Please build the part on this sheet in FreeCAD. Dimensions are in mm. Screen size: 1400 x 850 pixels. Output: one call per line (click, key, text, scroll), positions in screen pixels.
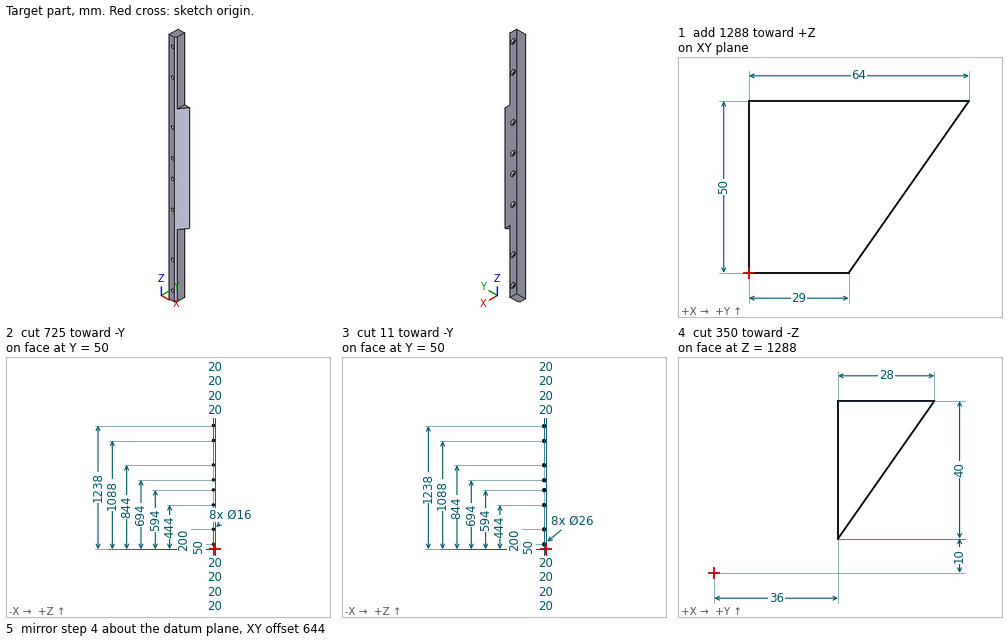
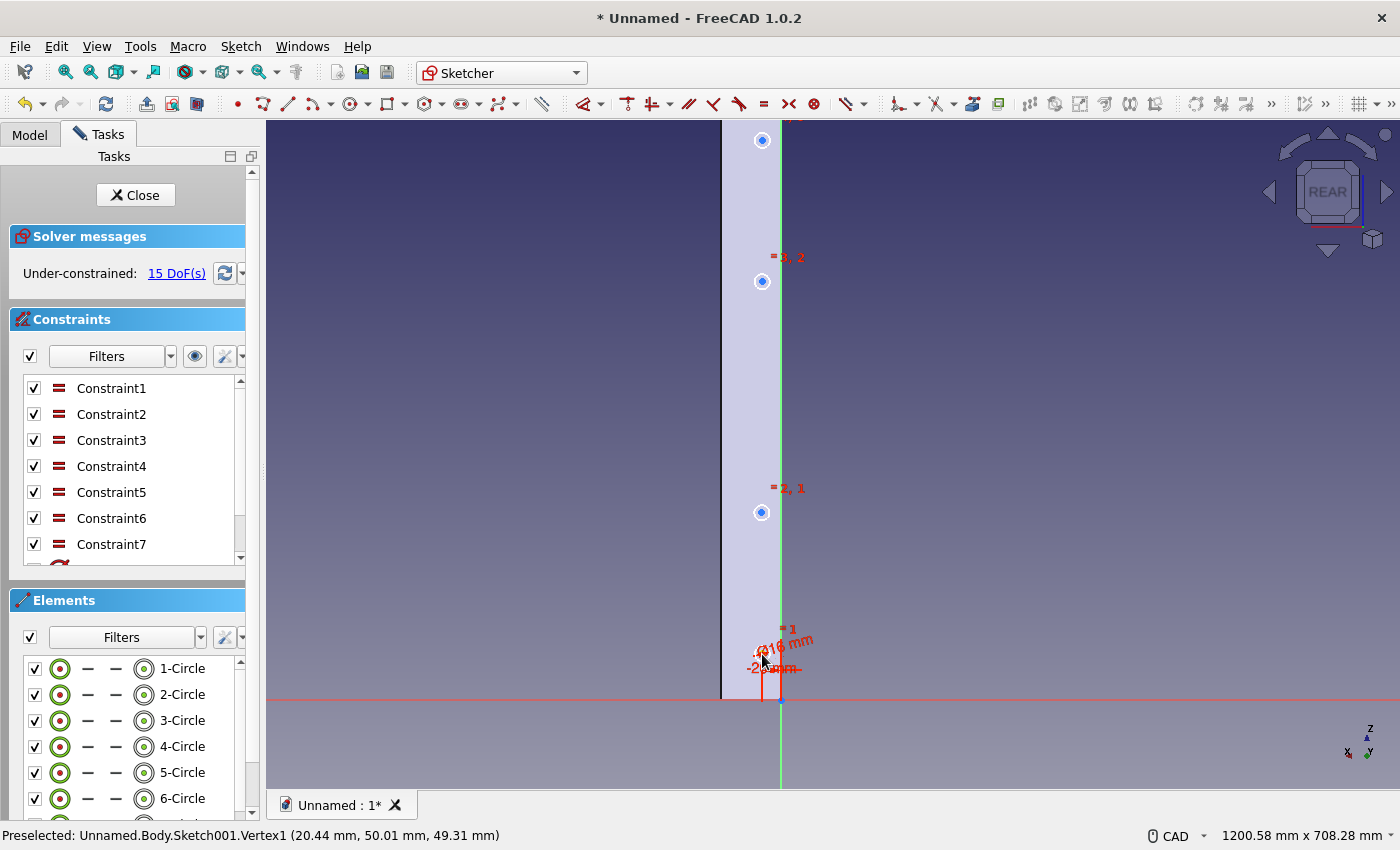
click(762, 654)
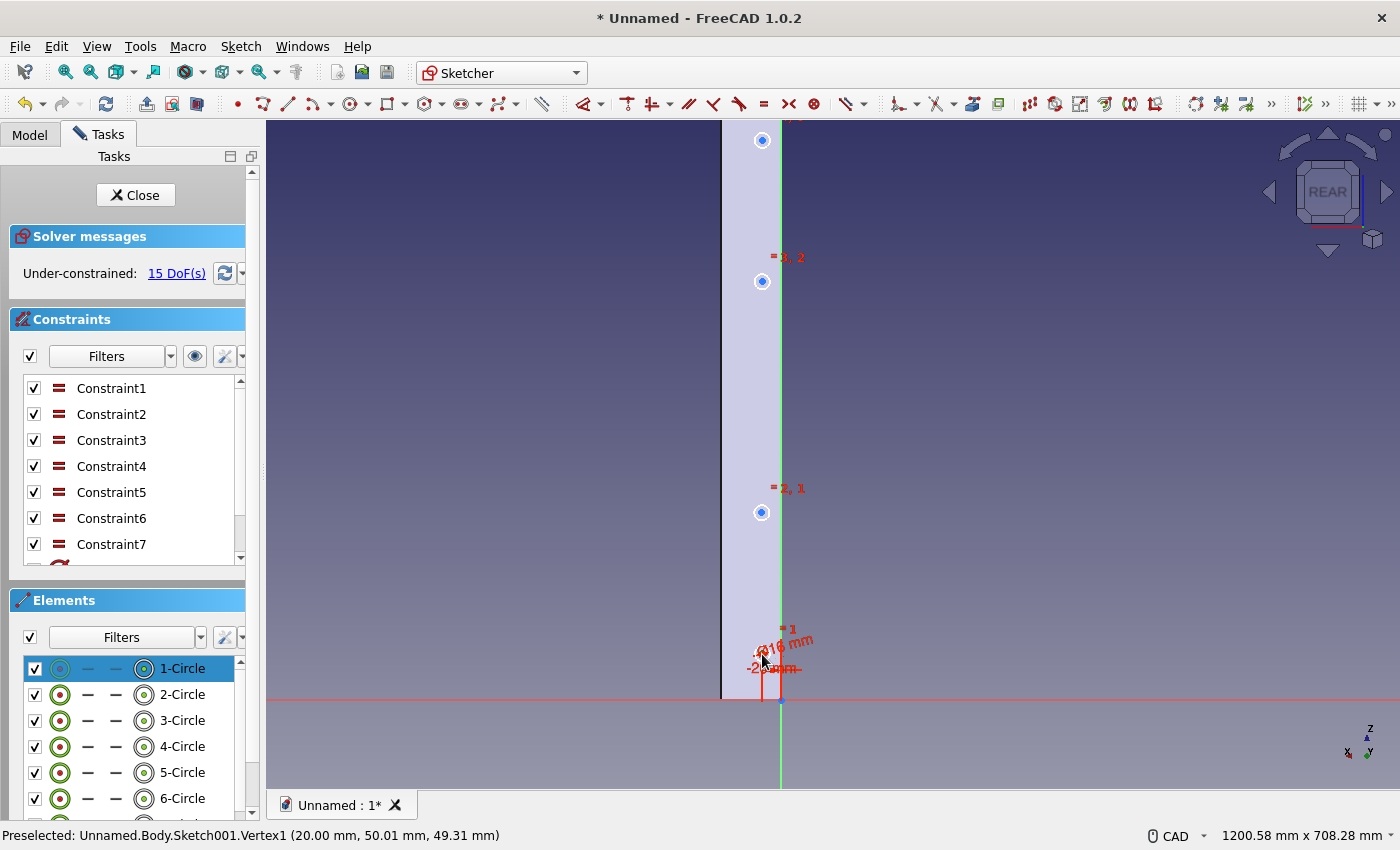
click(600, 104)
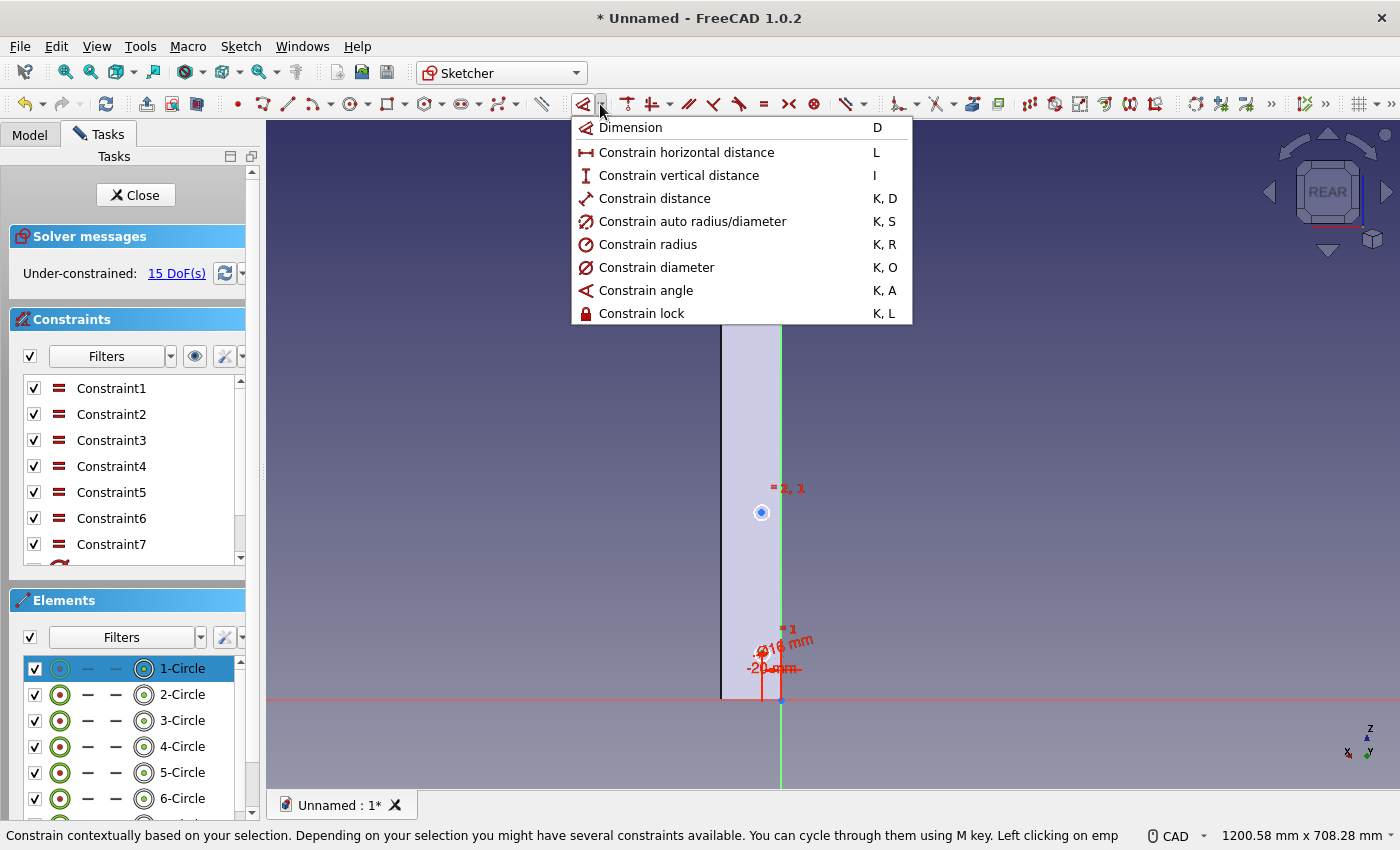
click(742, 176)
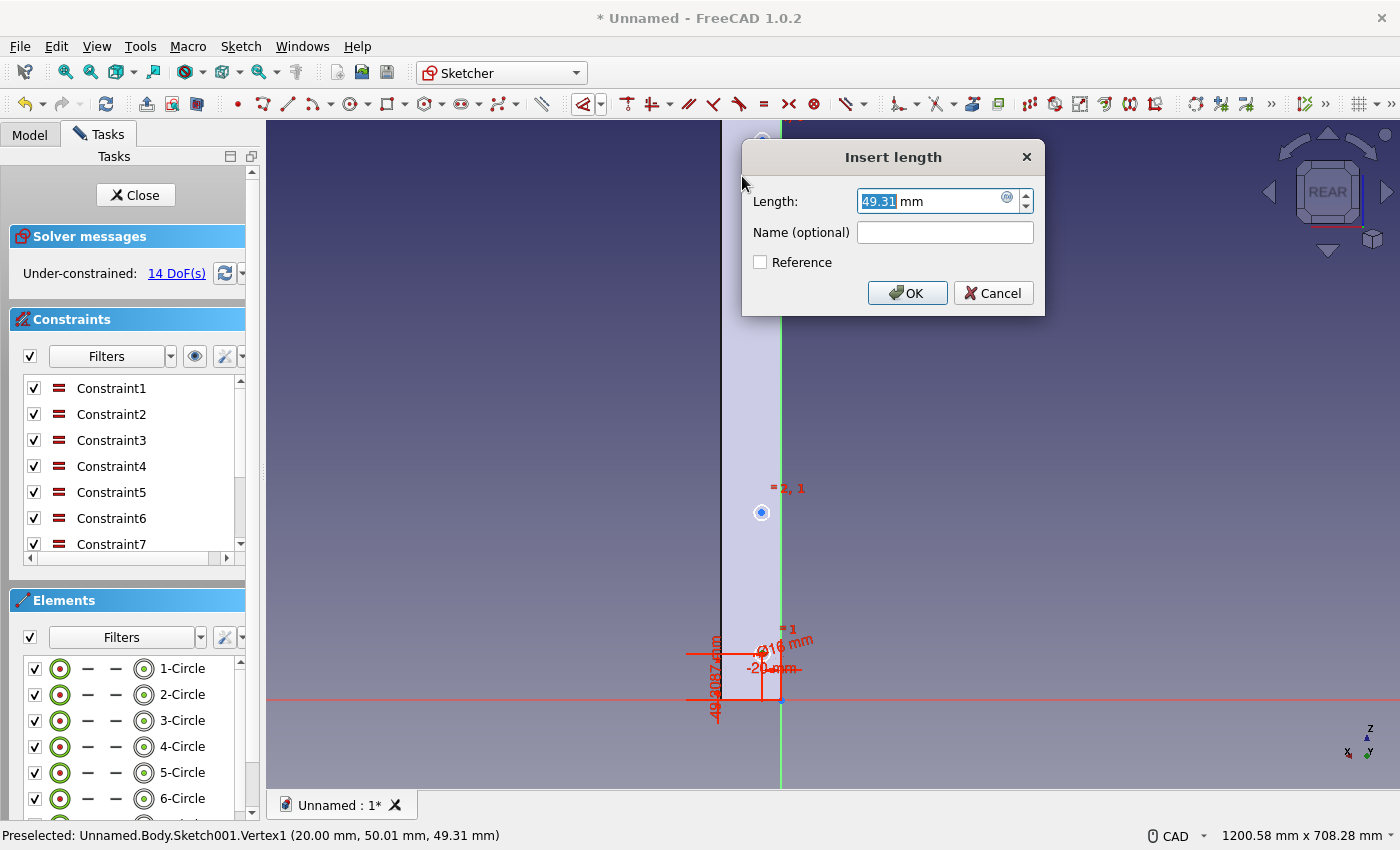
text(50)
key(Return)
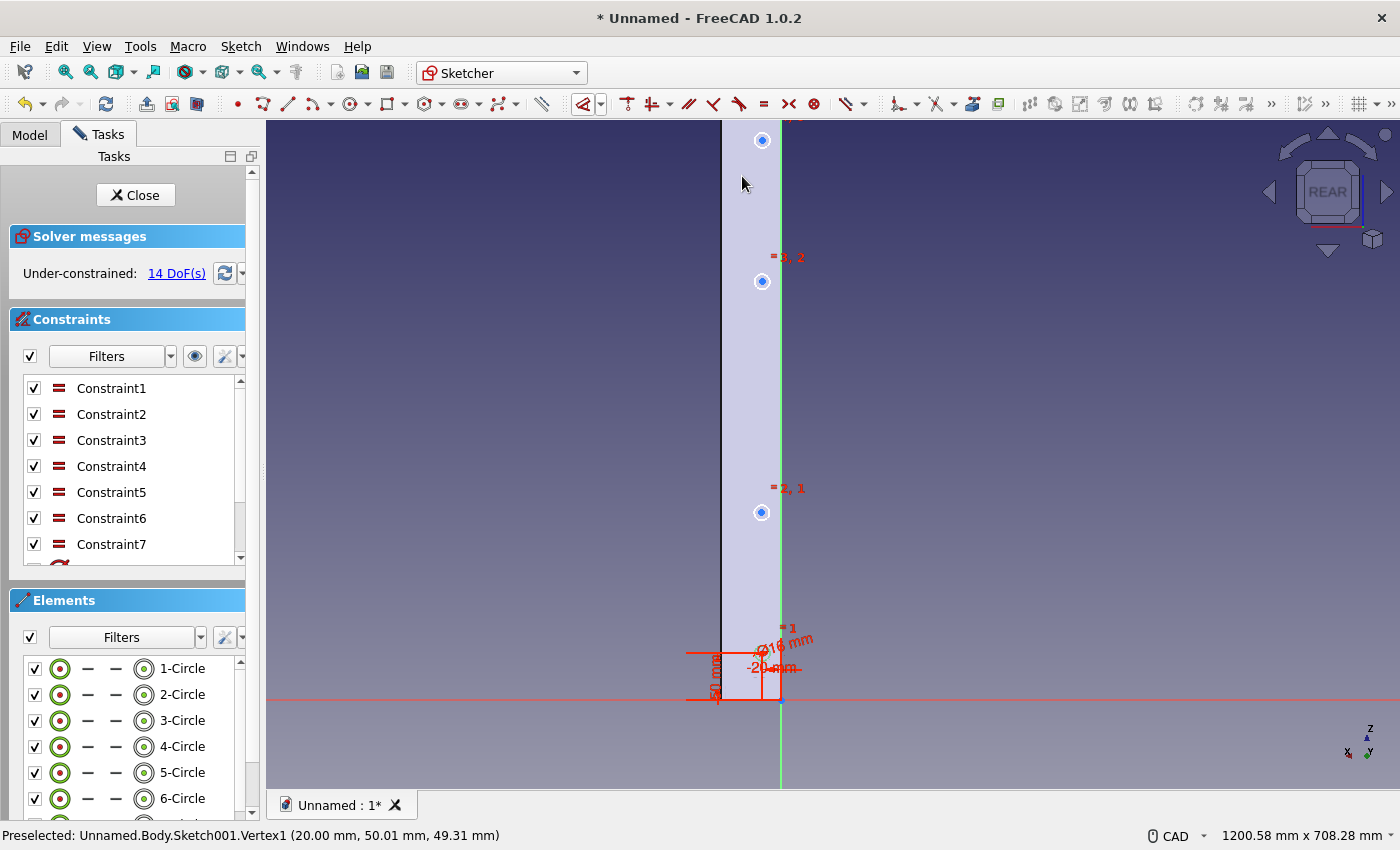
scroll(762, 513, up, 4)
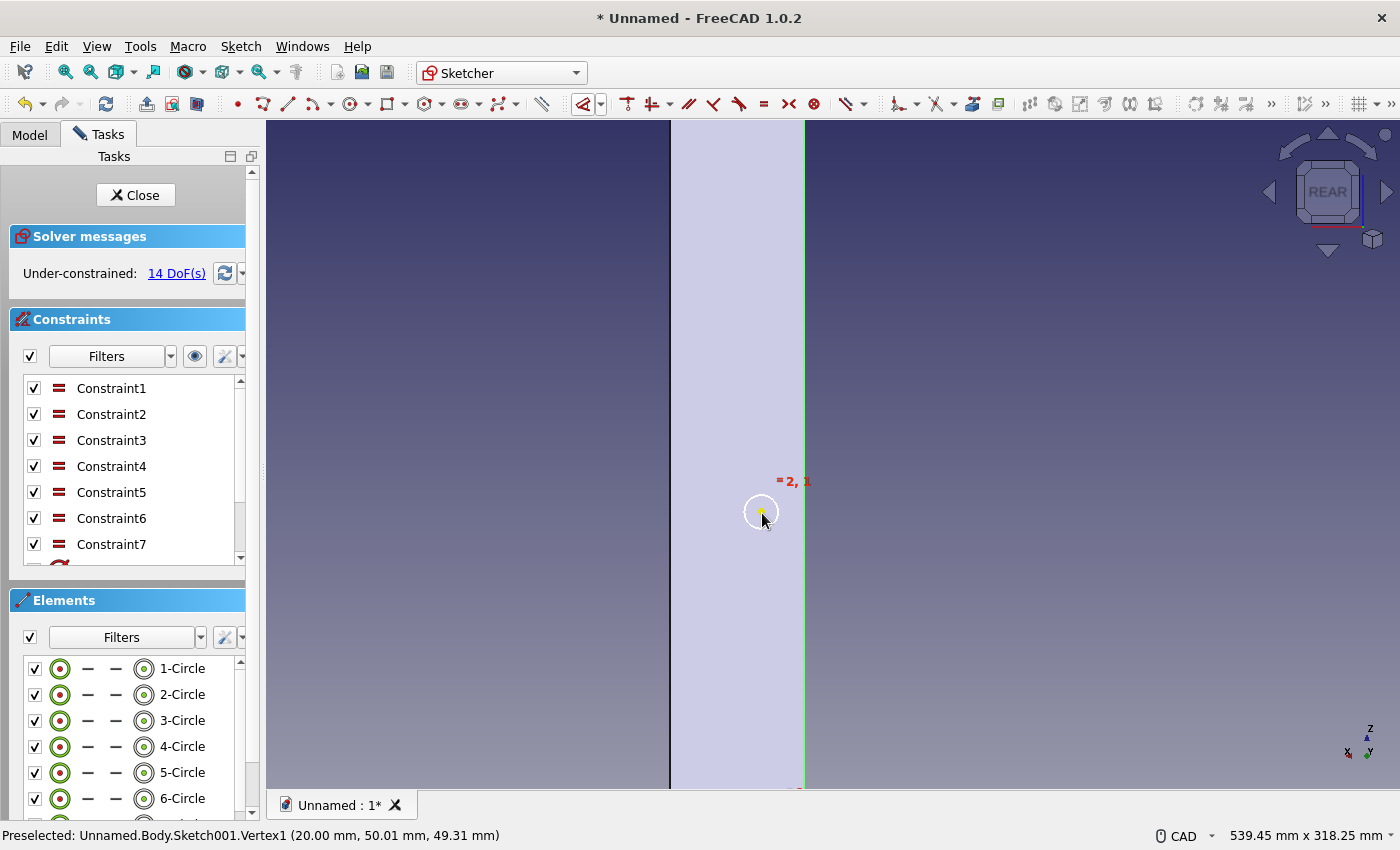
click(761, 512)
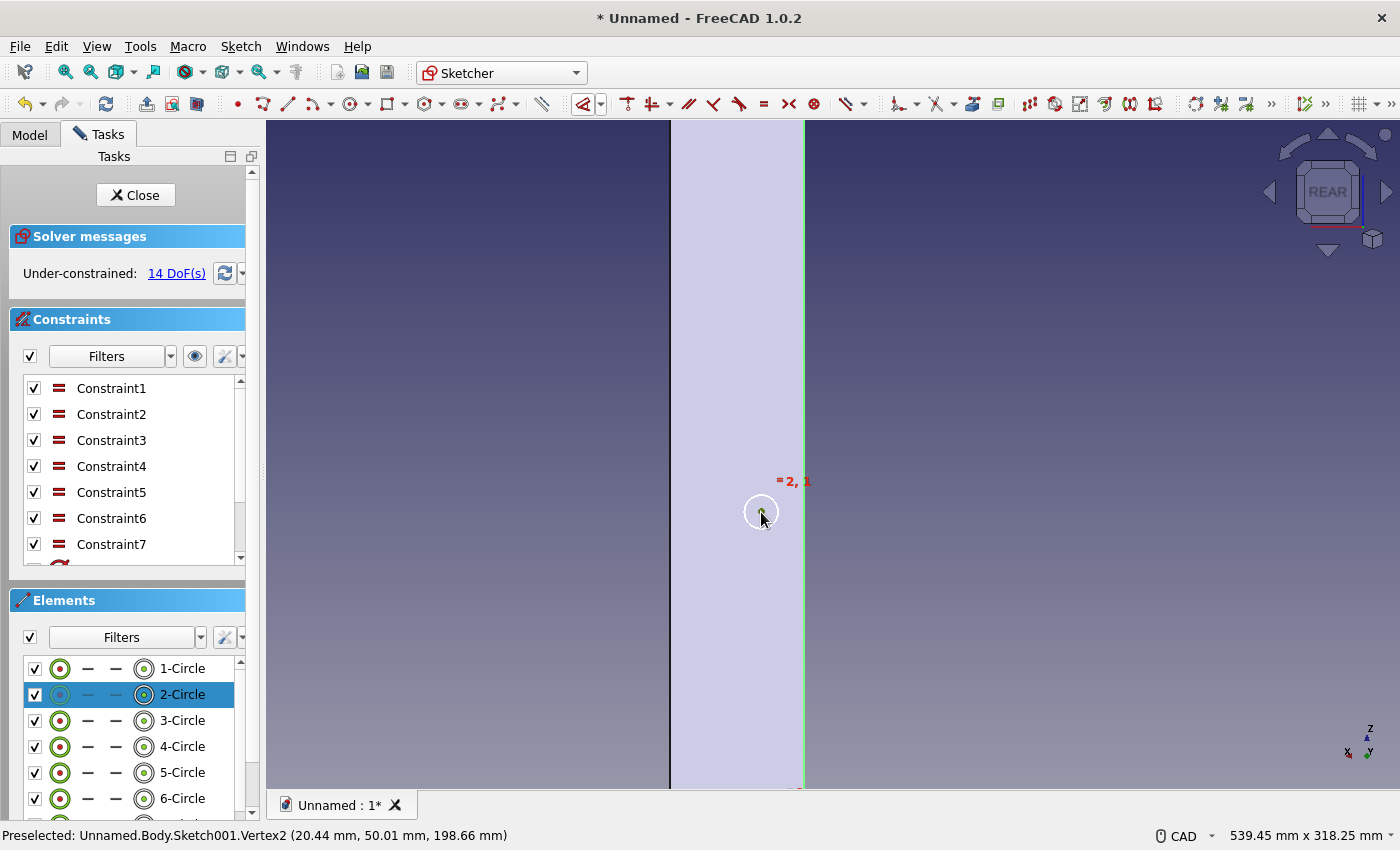
key(l)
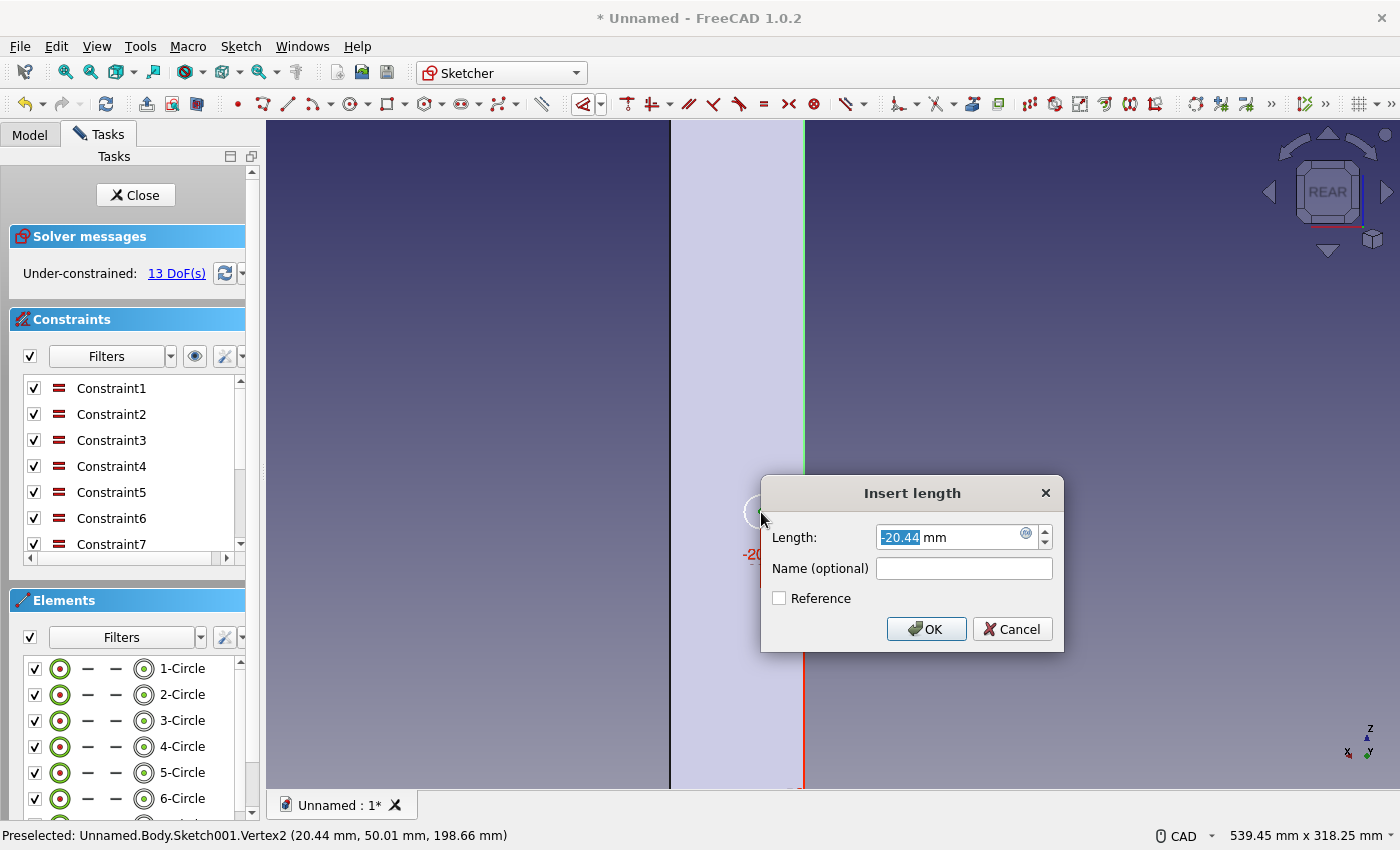
text(-20)
key(Return)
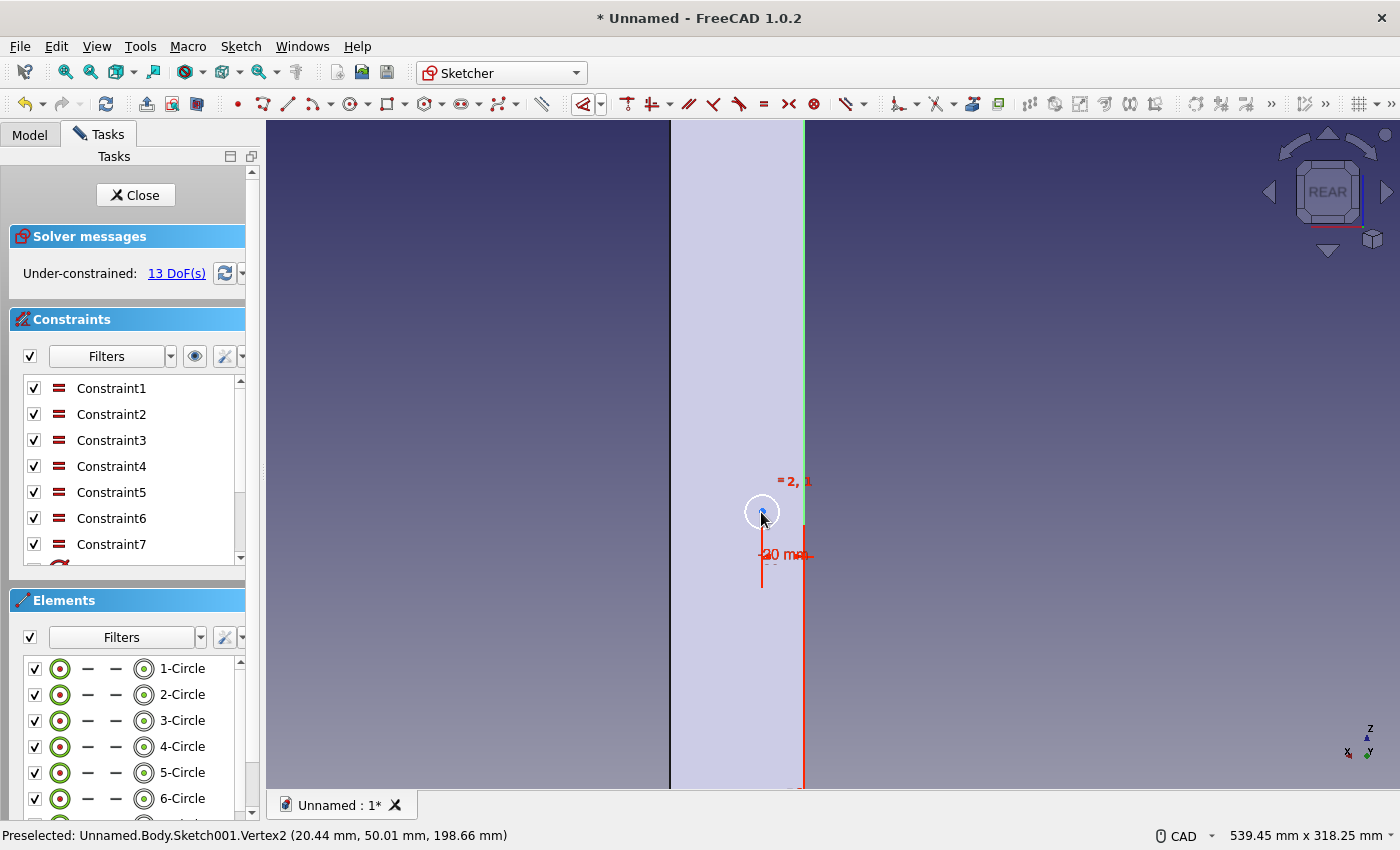
scroll(762, 620, down, 9)